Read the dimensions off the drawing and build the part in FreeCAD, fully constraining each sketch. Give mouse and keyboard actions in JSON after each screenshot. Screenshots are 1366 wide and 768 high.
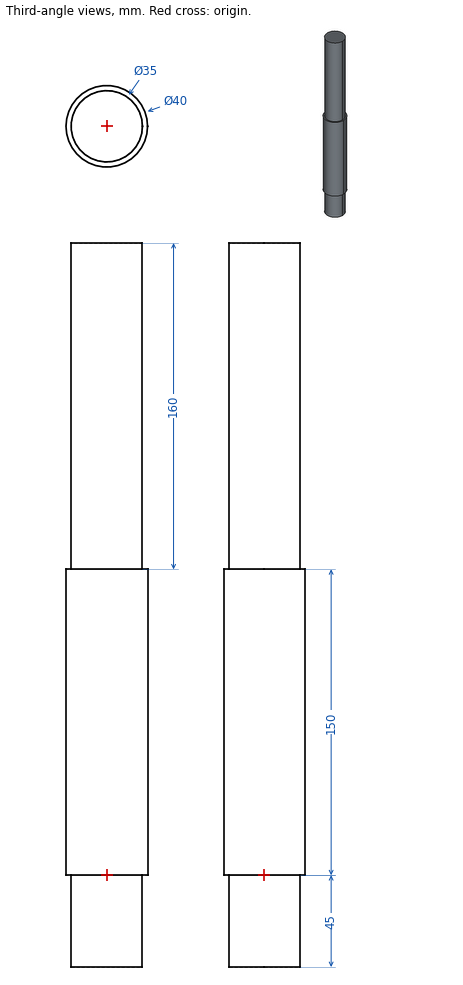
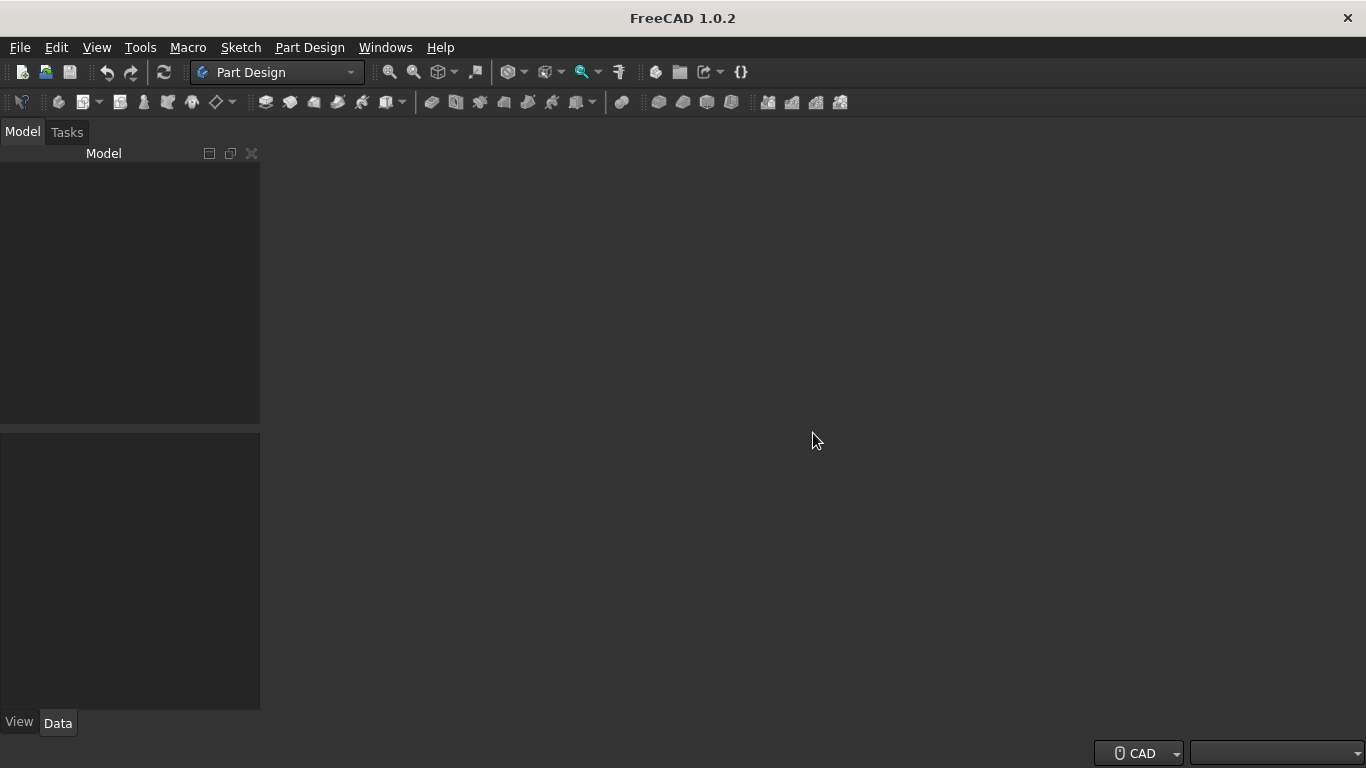
{"action": "key", "text": "ctrl+n"}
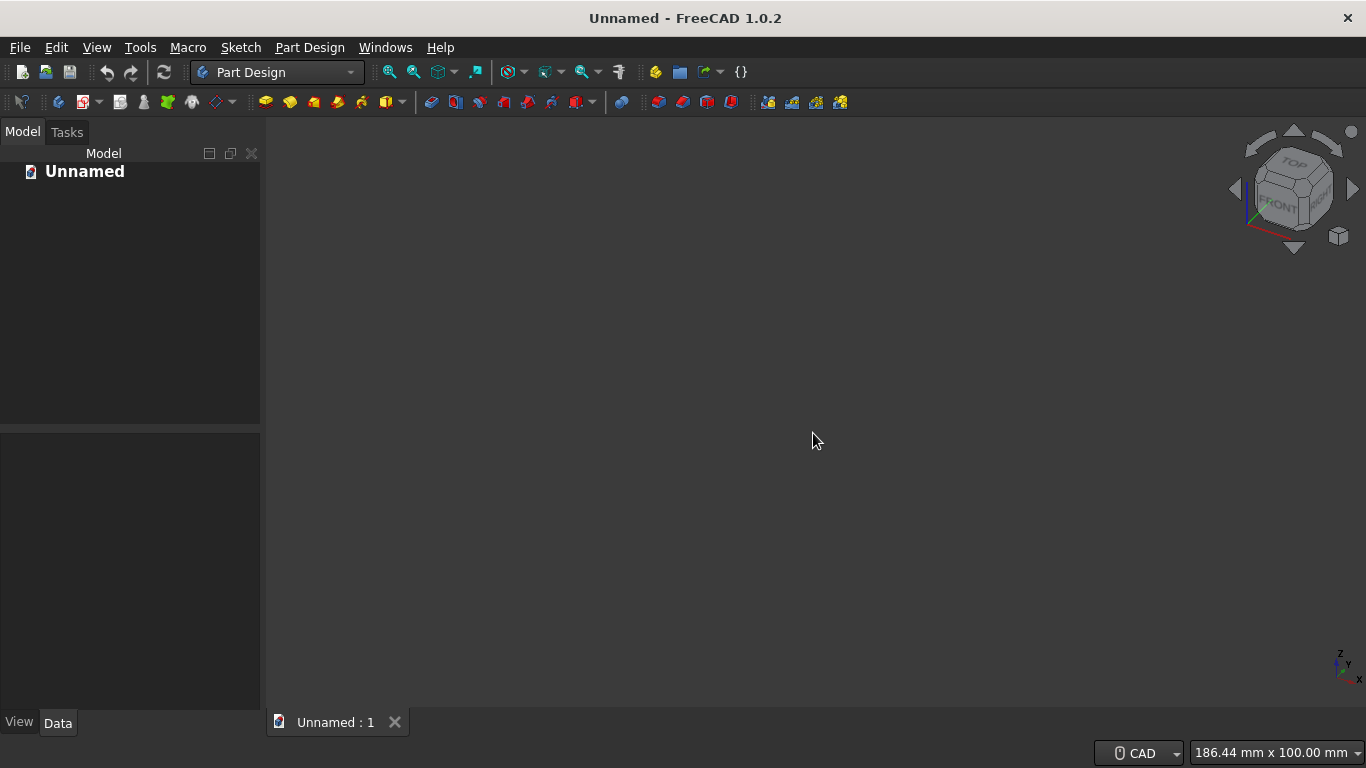
{"action": "left_click", "coordinate": [84, 102]}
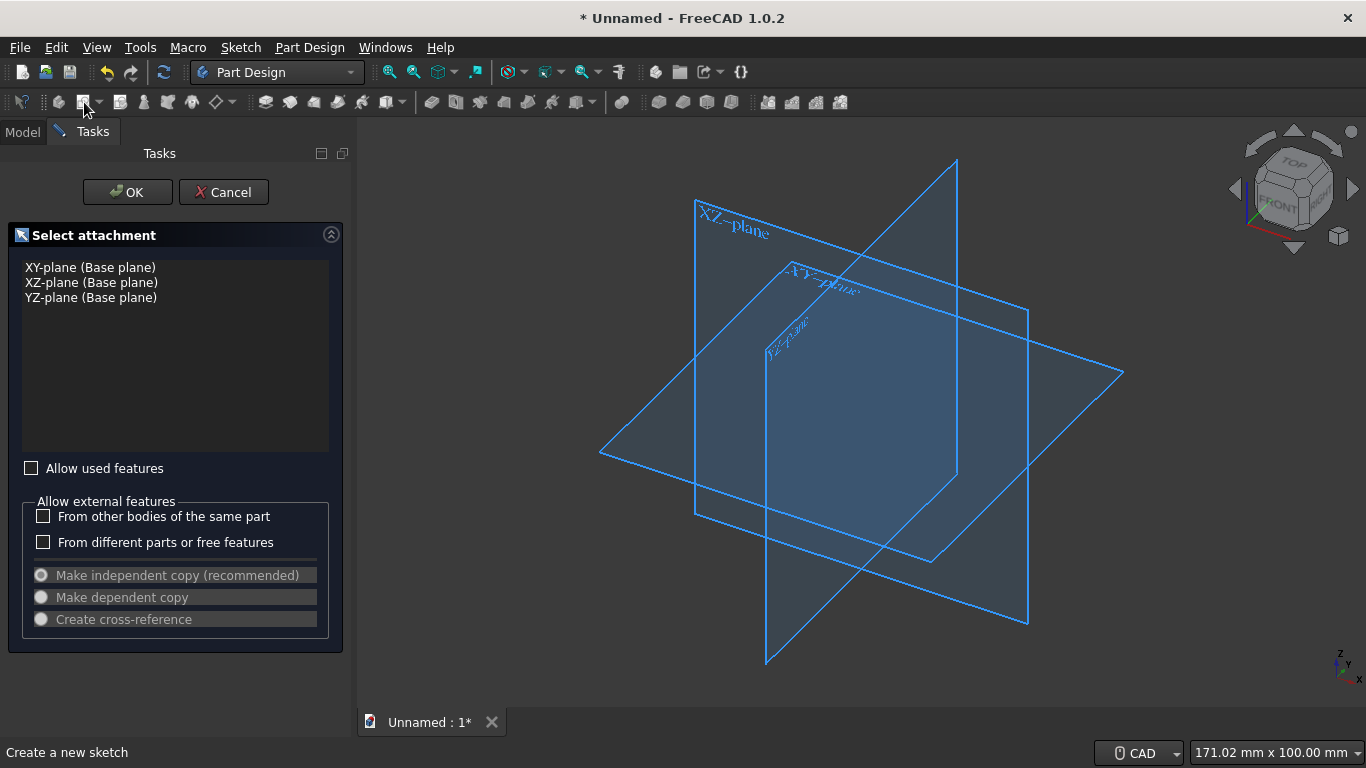
{"action": "left_click", "coordinate": [82, 268]}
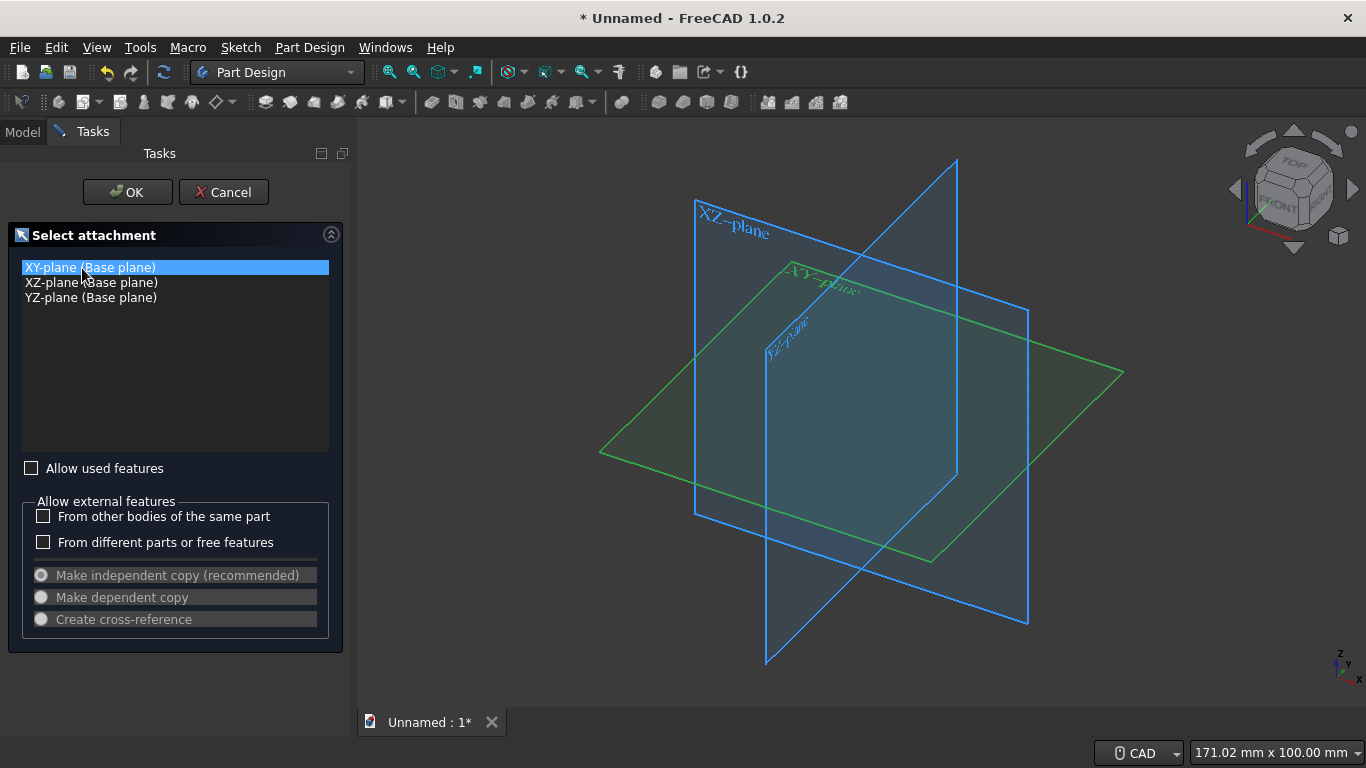
{"action": "left_click", "coordinate": [128, 192]}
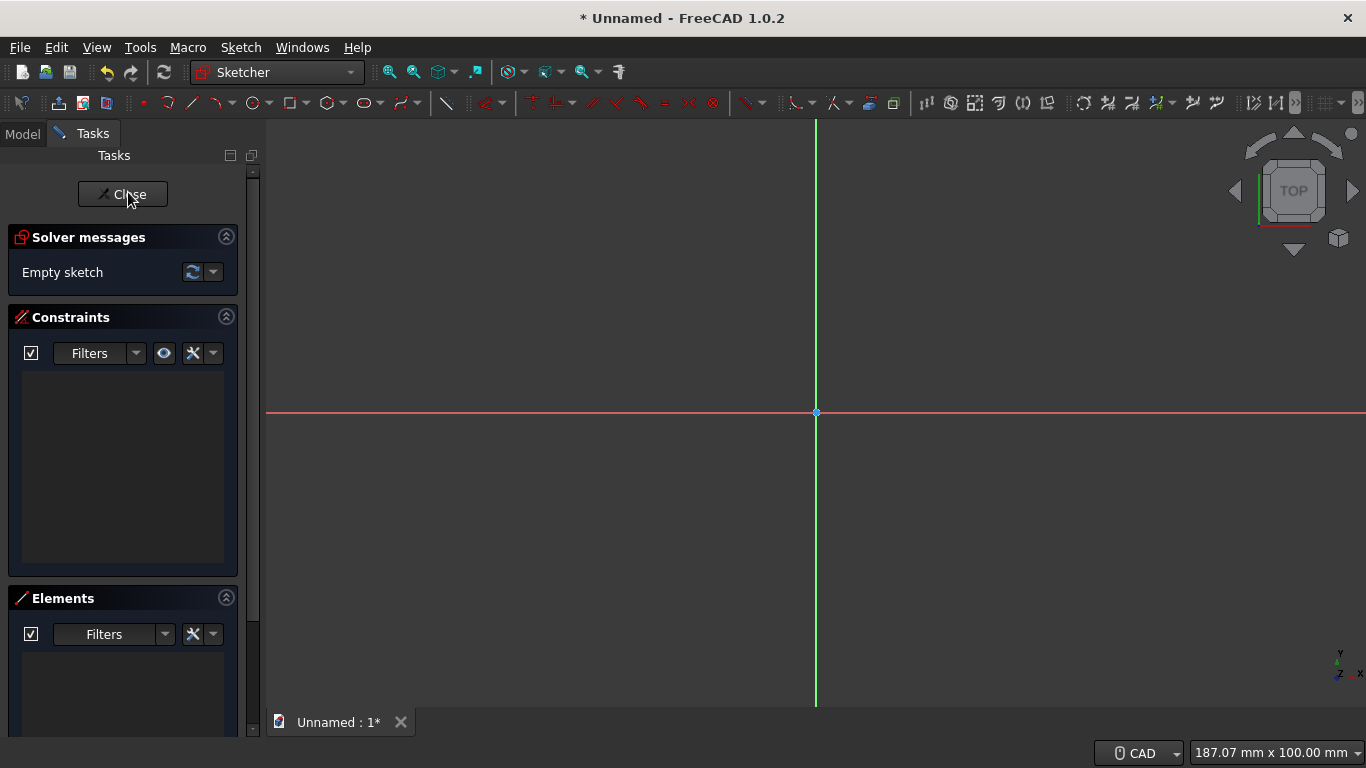
{"action": "scroll", "coordinate": [955, 413], "scroll_direction": "up", "scroll_amount": 2}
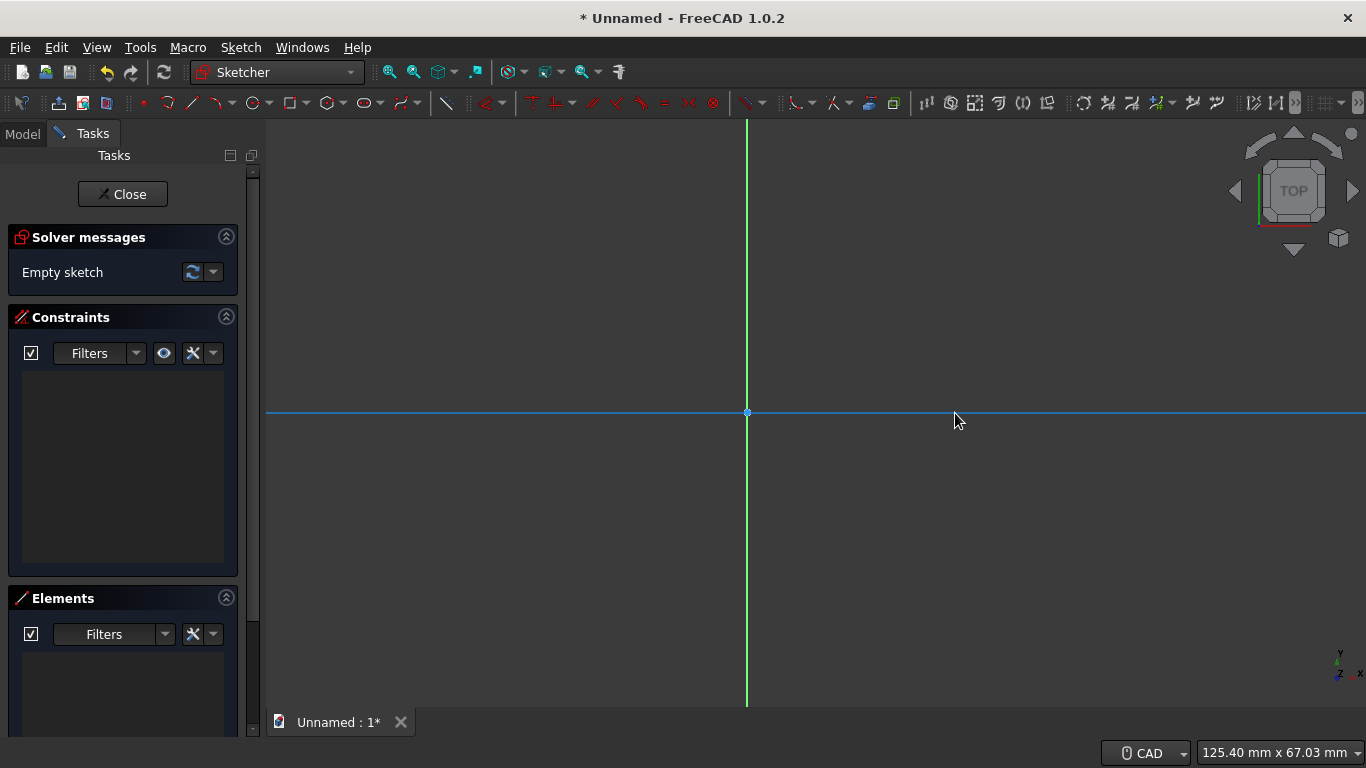
{"action": "key", "text": "g c"}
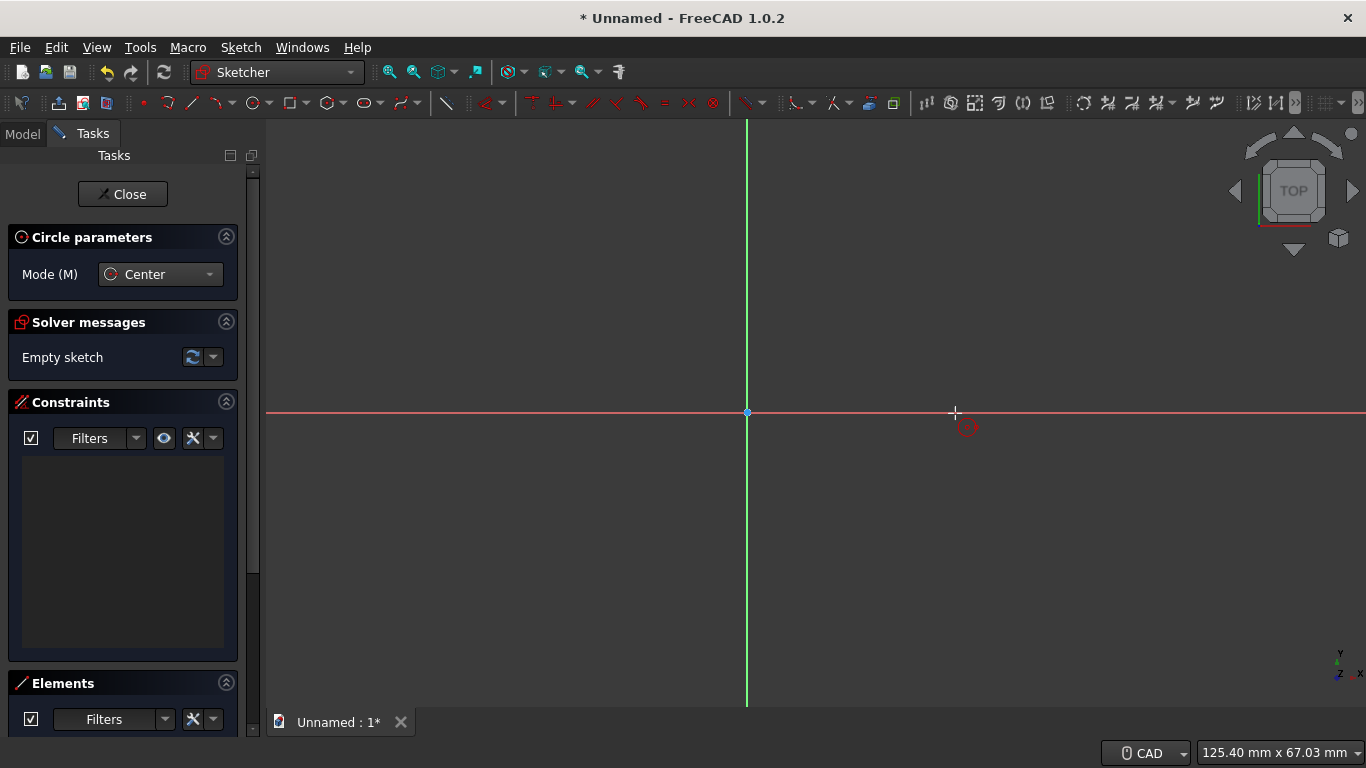
{"action": "left_click", "coordinate": [747, 413]}
{"action": "mouse_move", "coordinate": [871, 289]}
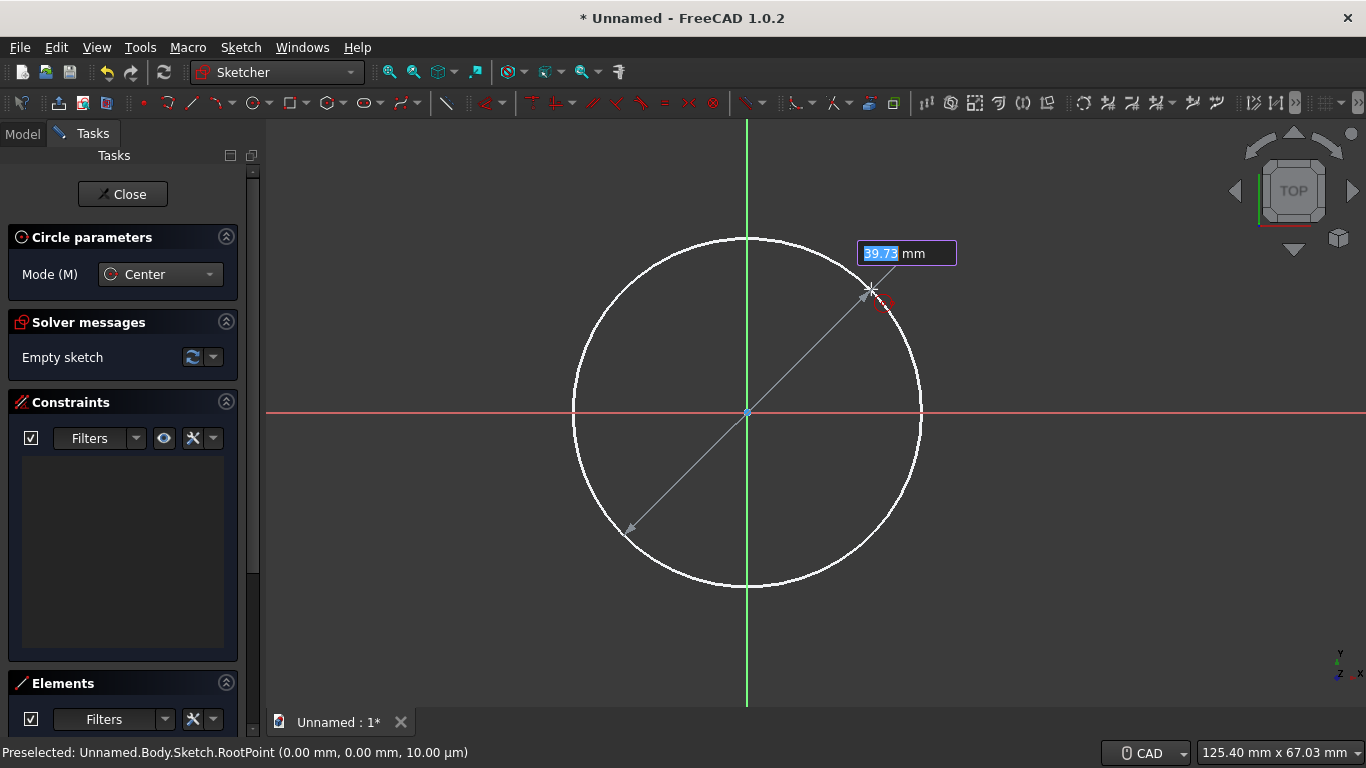
{"action": "type", "text": "40"}
{"action": "key", "text": "Return"}
{"action": "key", "text": "Escape"}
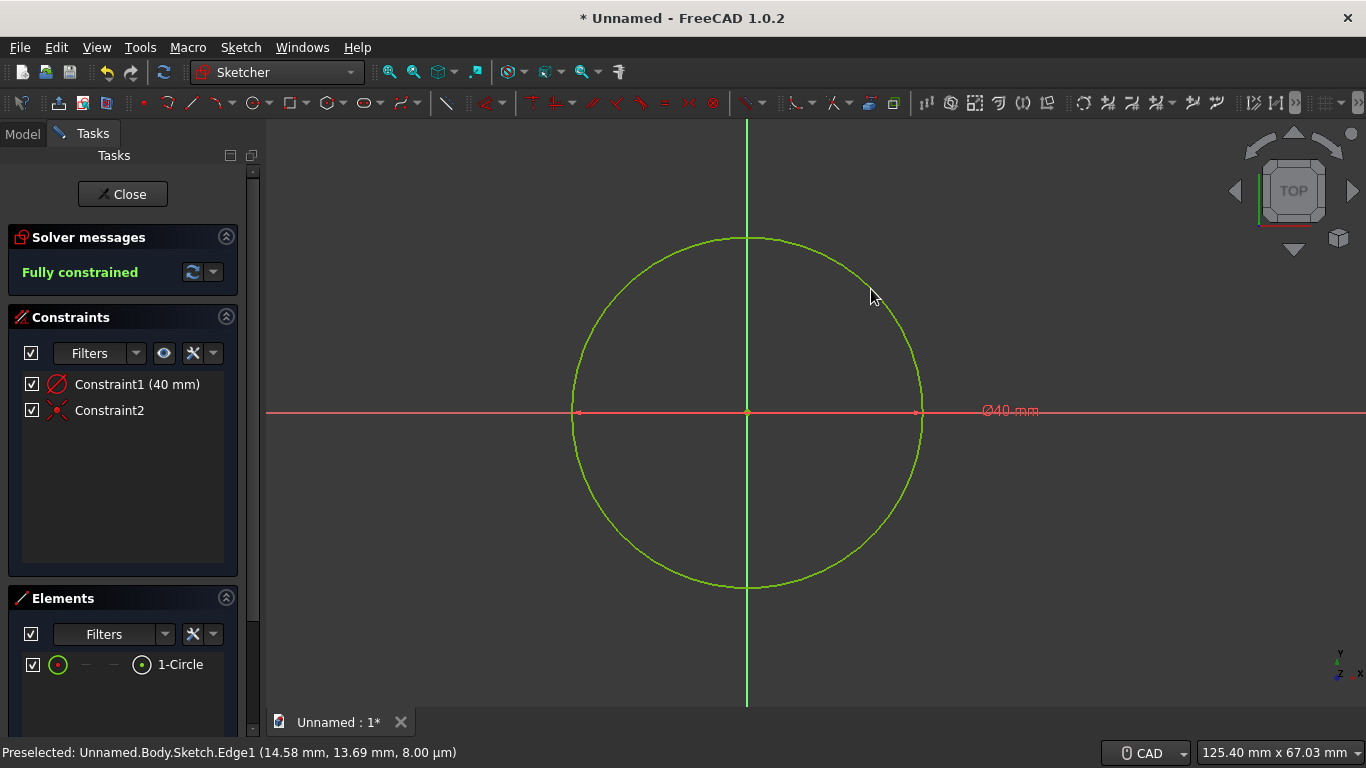
{"action": "left_click", "coordinate": [123, 194]}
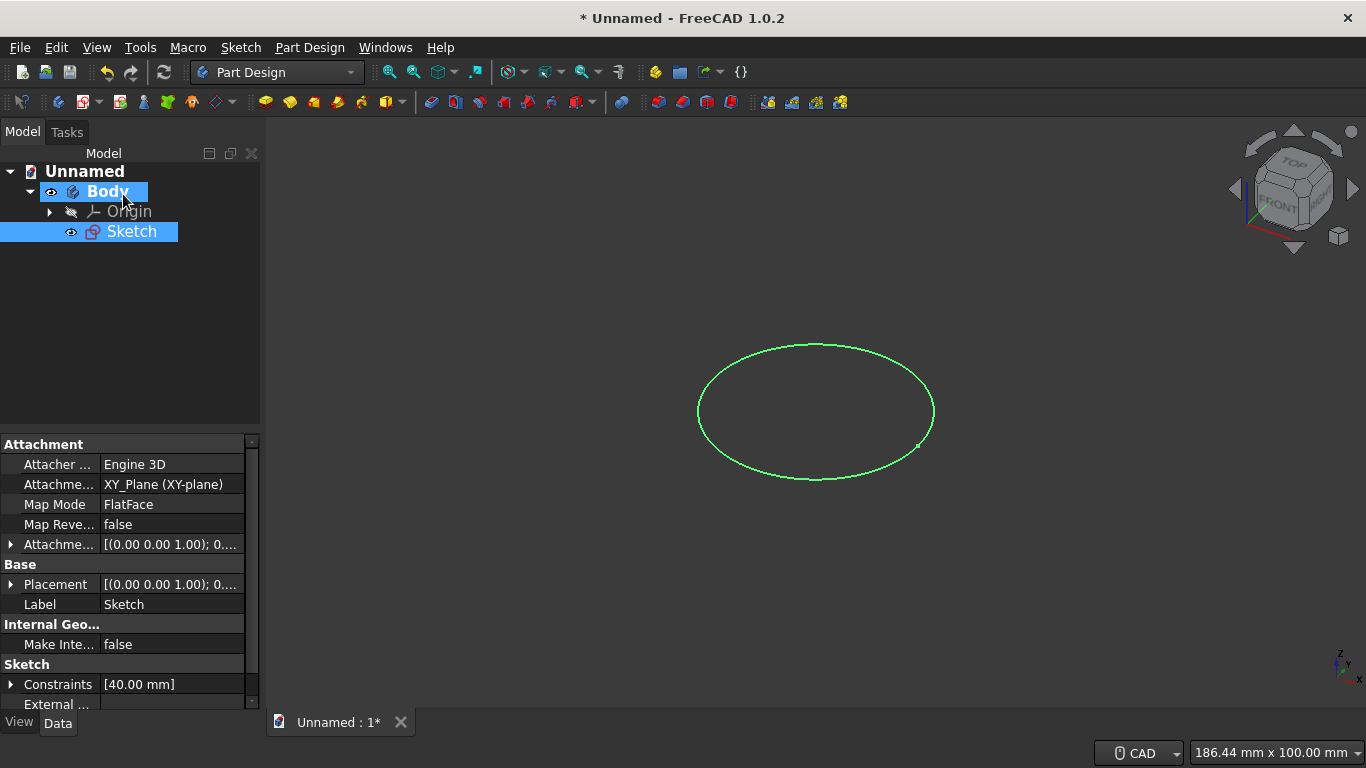
{"action": "left_click", "coordinate": [266, 102]}